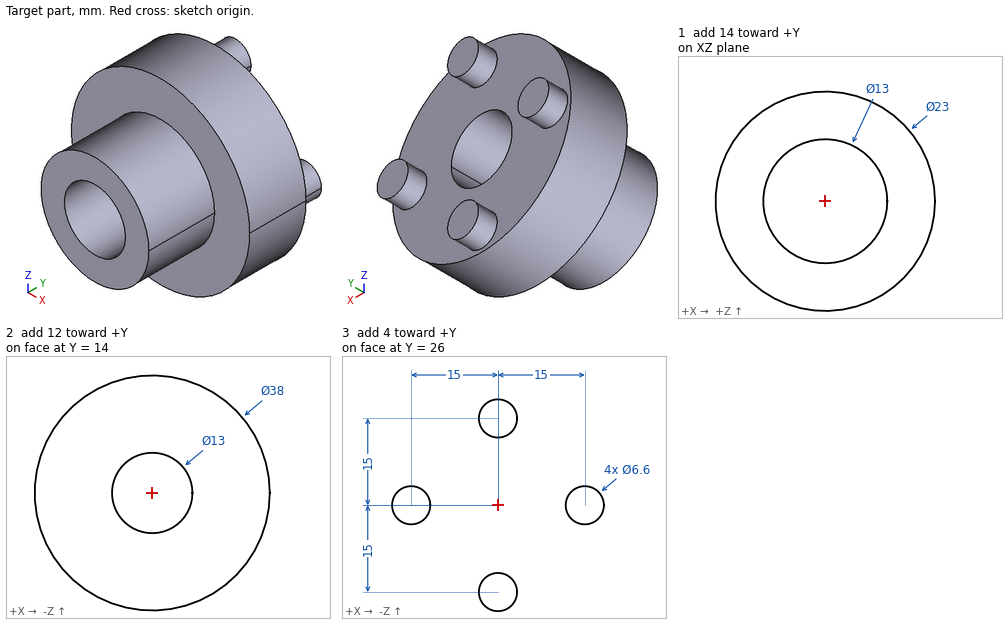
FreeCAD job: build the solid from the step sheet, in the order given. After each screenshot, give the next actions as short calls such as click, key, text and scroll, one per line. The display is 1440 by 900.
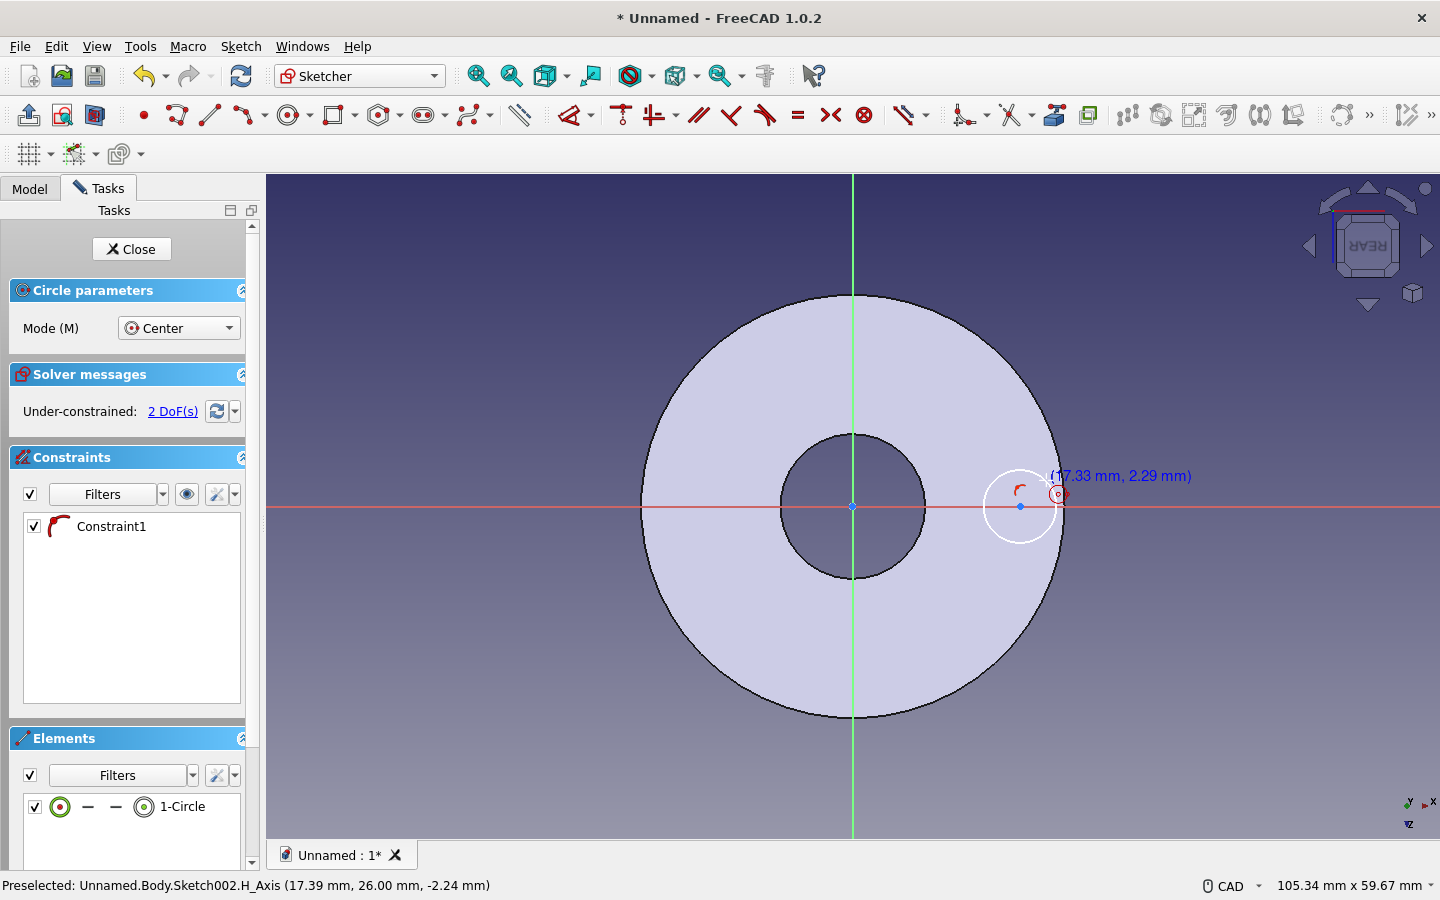
click(853, 339)
click(879, 313)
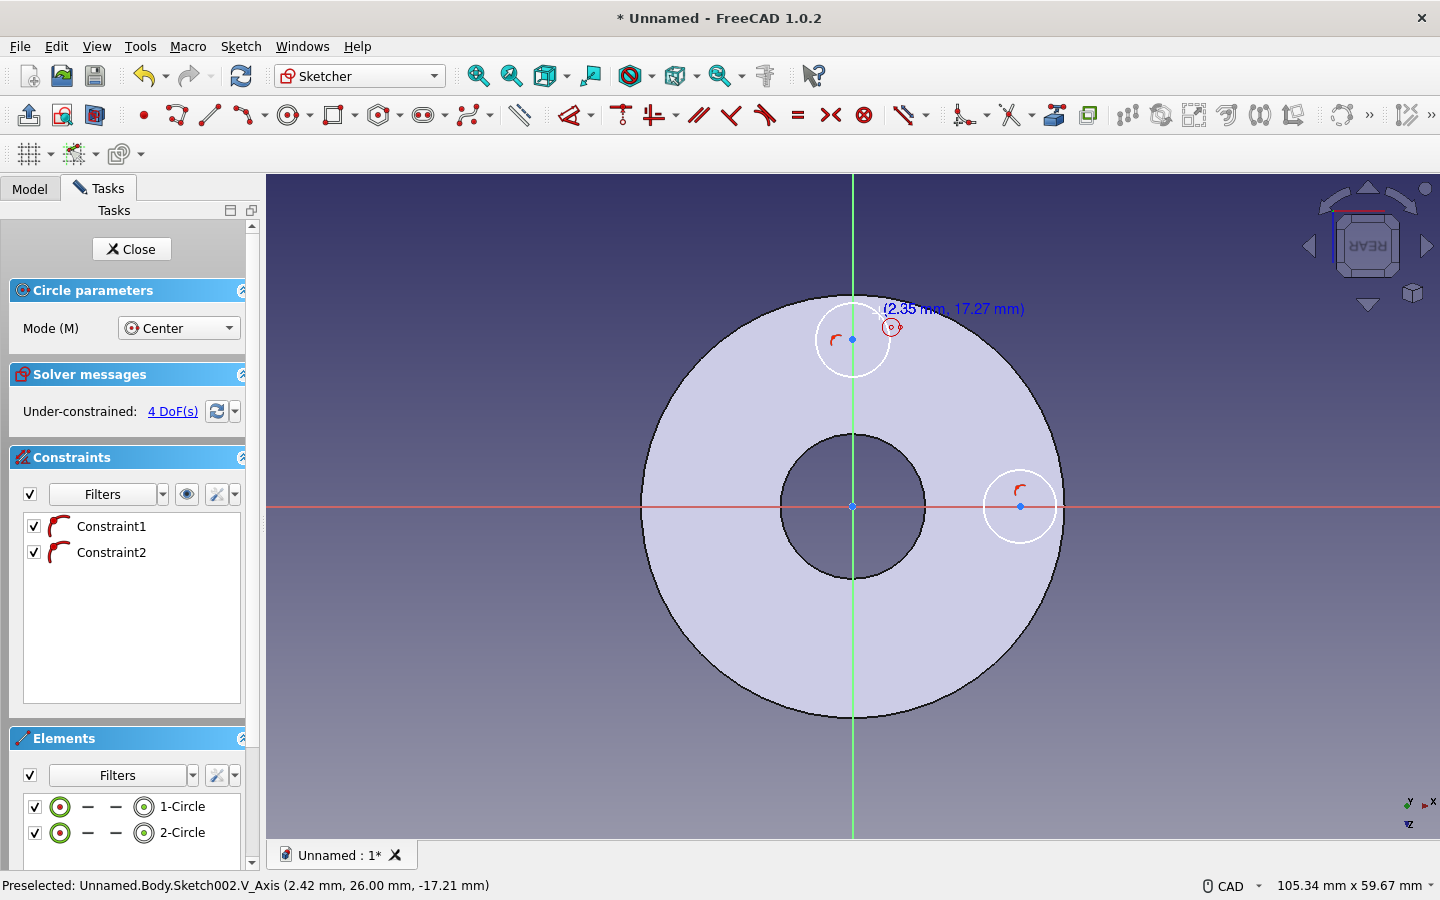
click(853, 674)
click(879, 648)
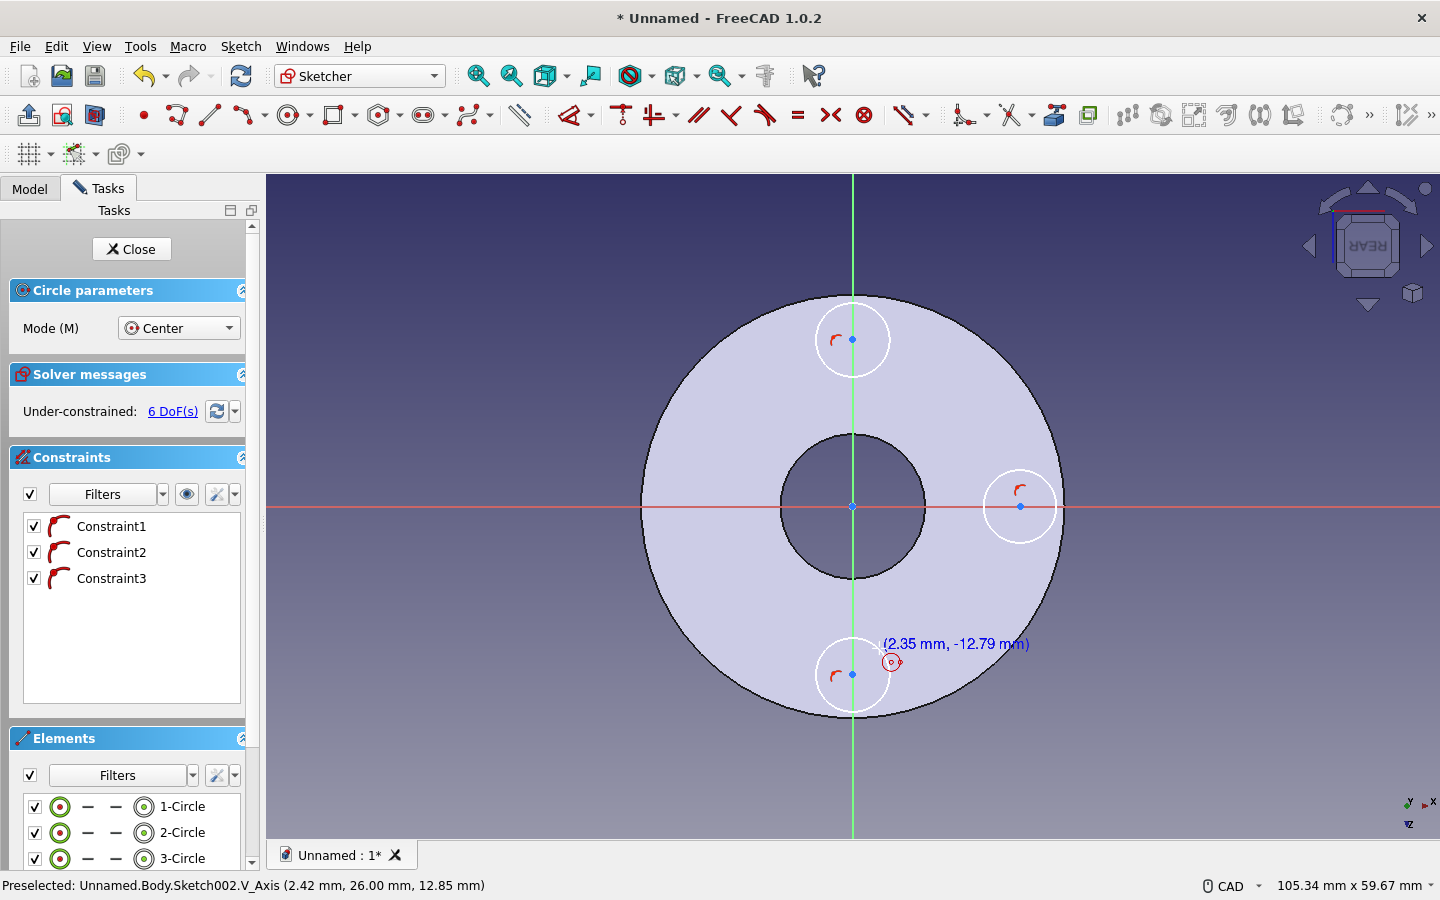
click(686, 506)
click(712, 480)
key(Escape)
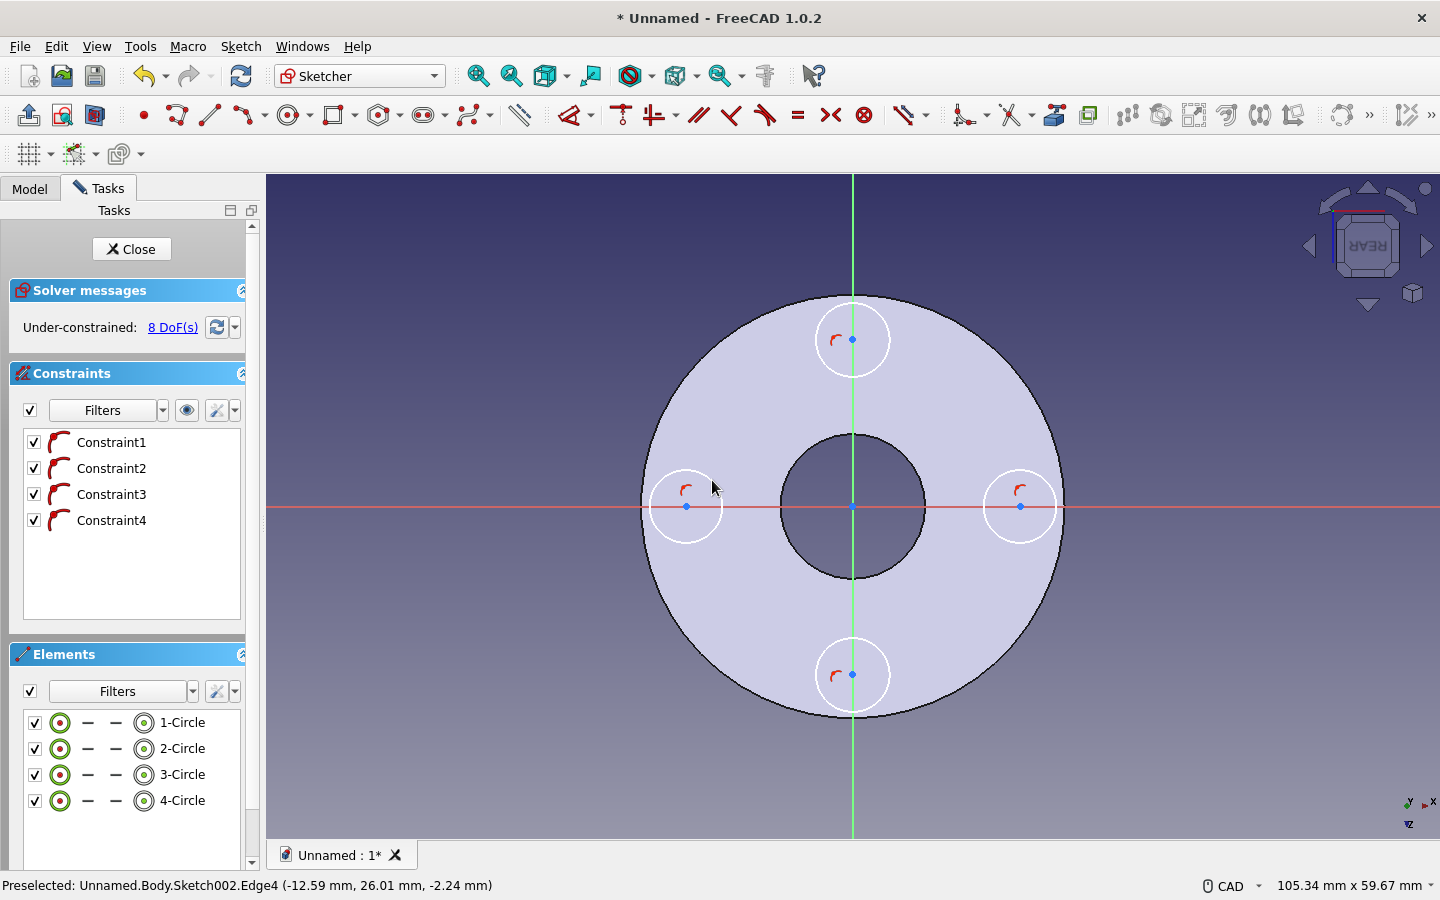
click(1046, 481)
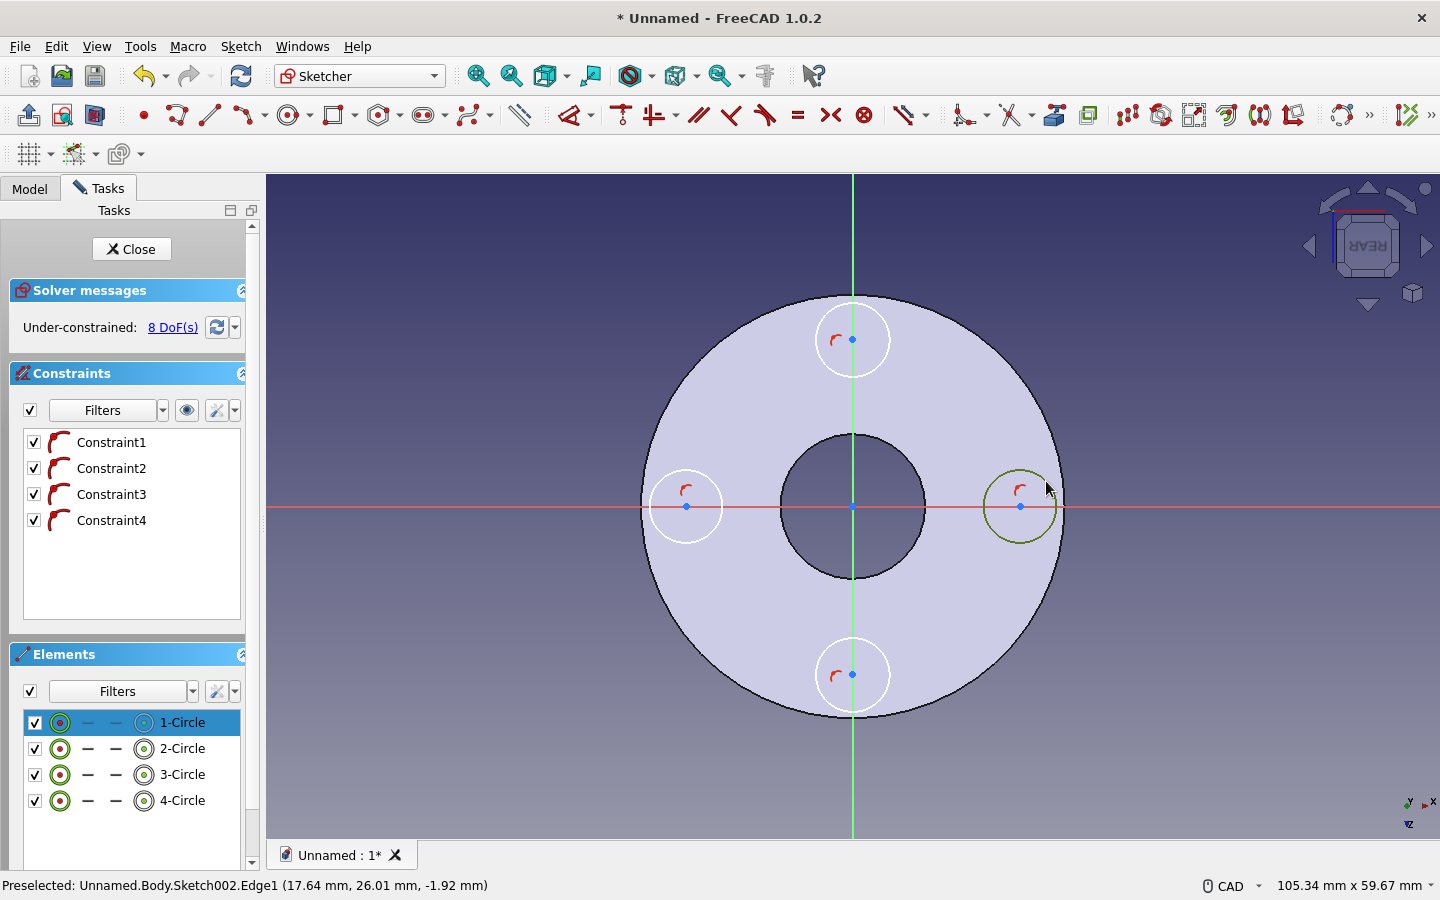
click(879, 314)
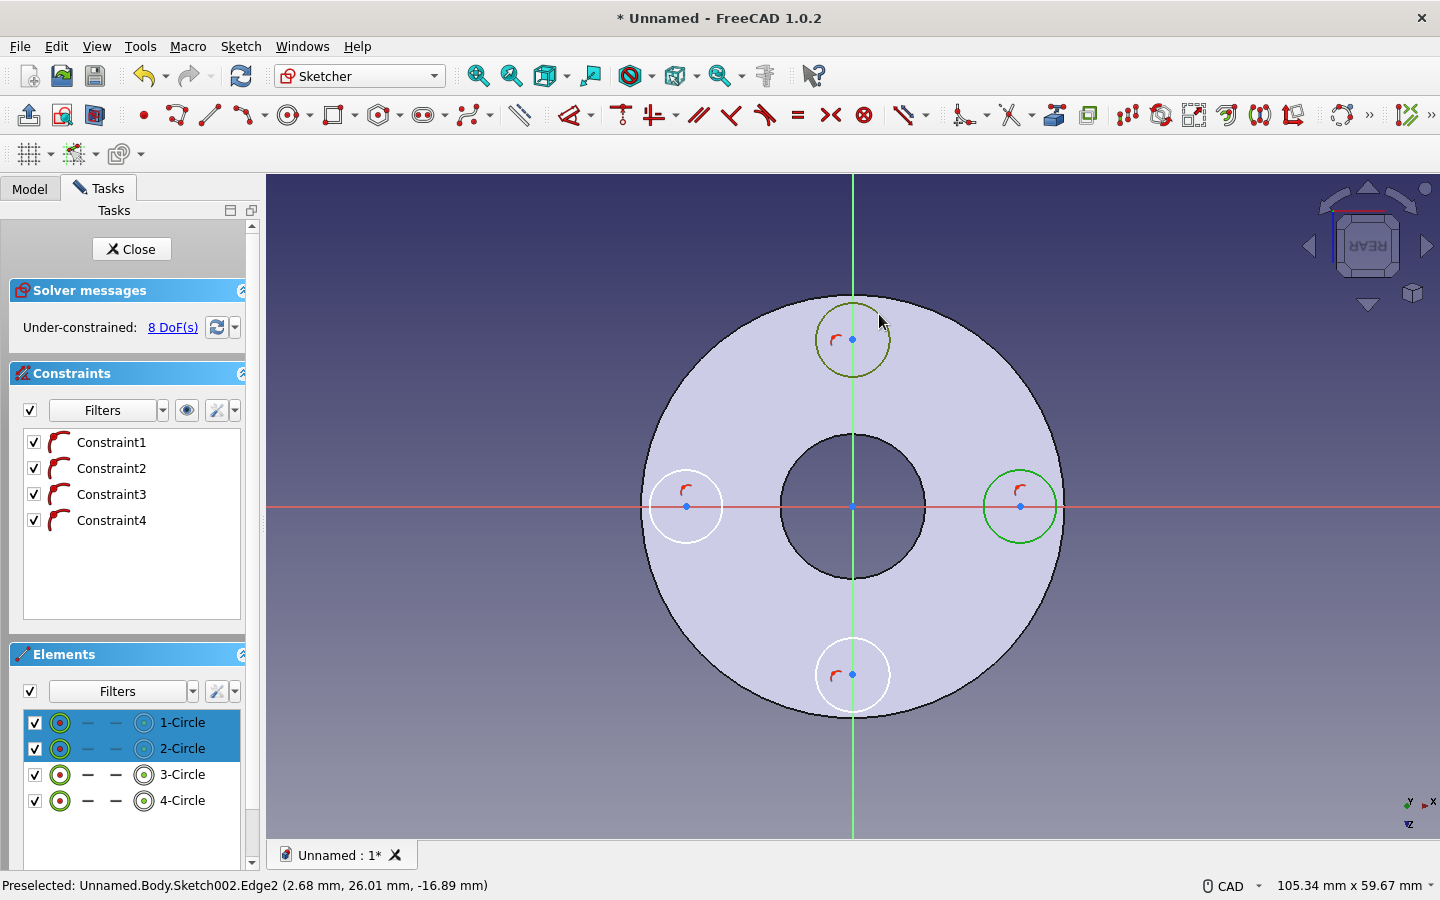
click(879, 649)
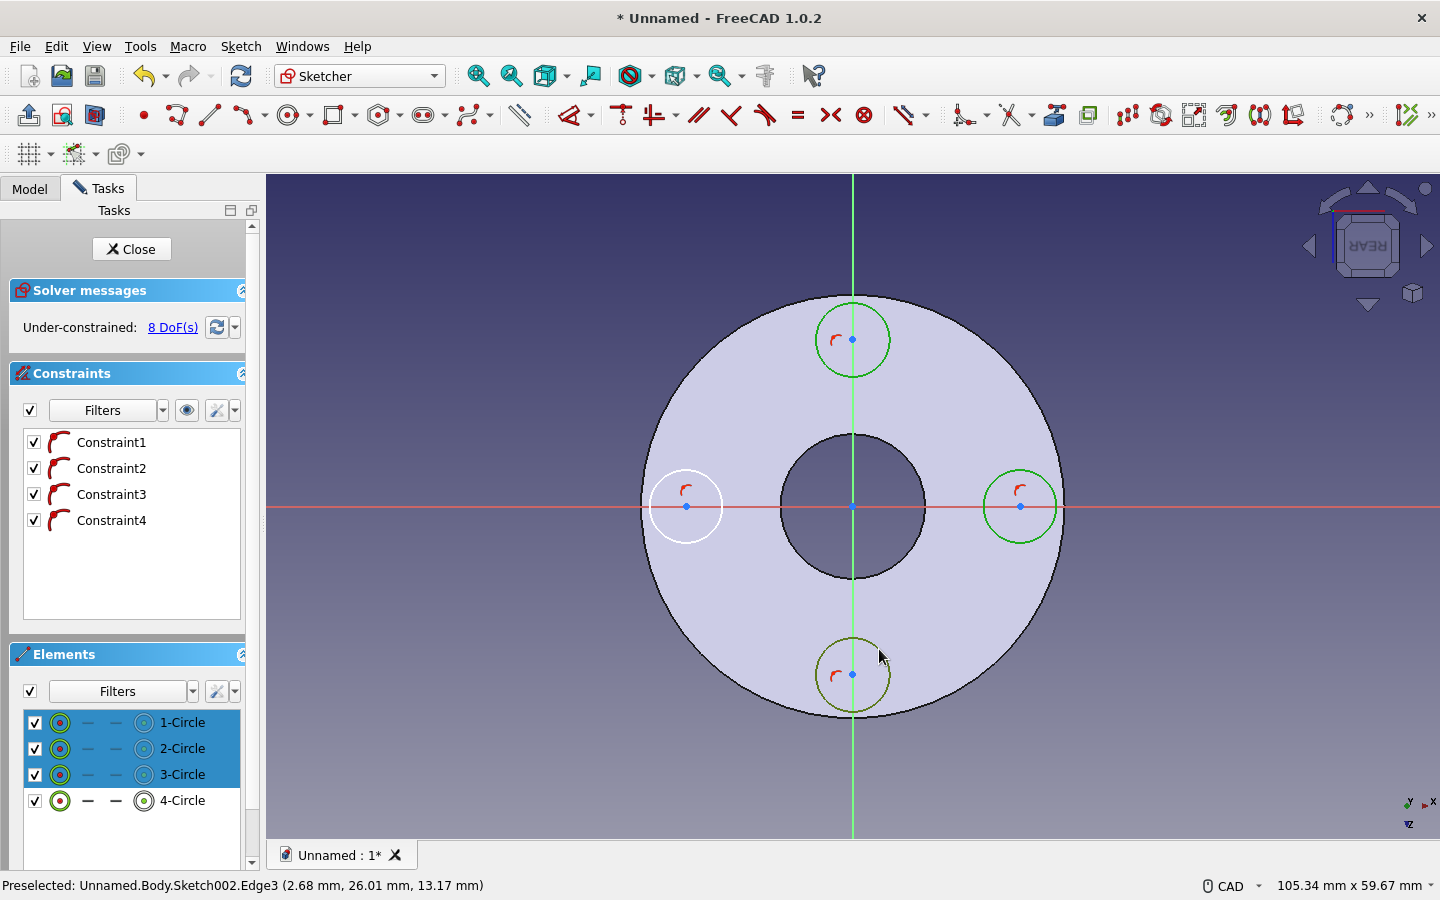
click(712, 481)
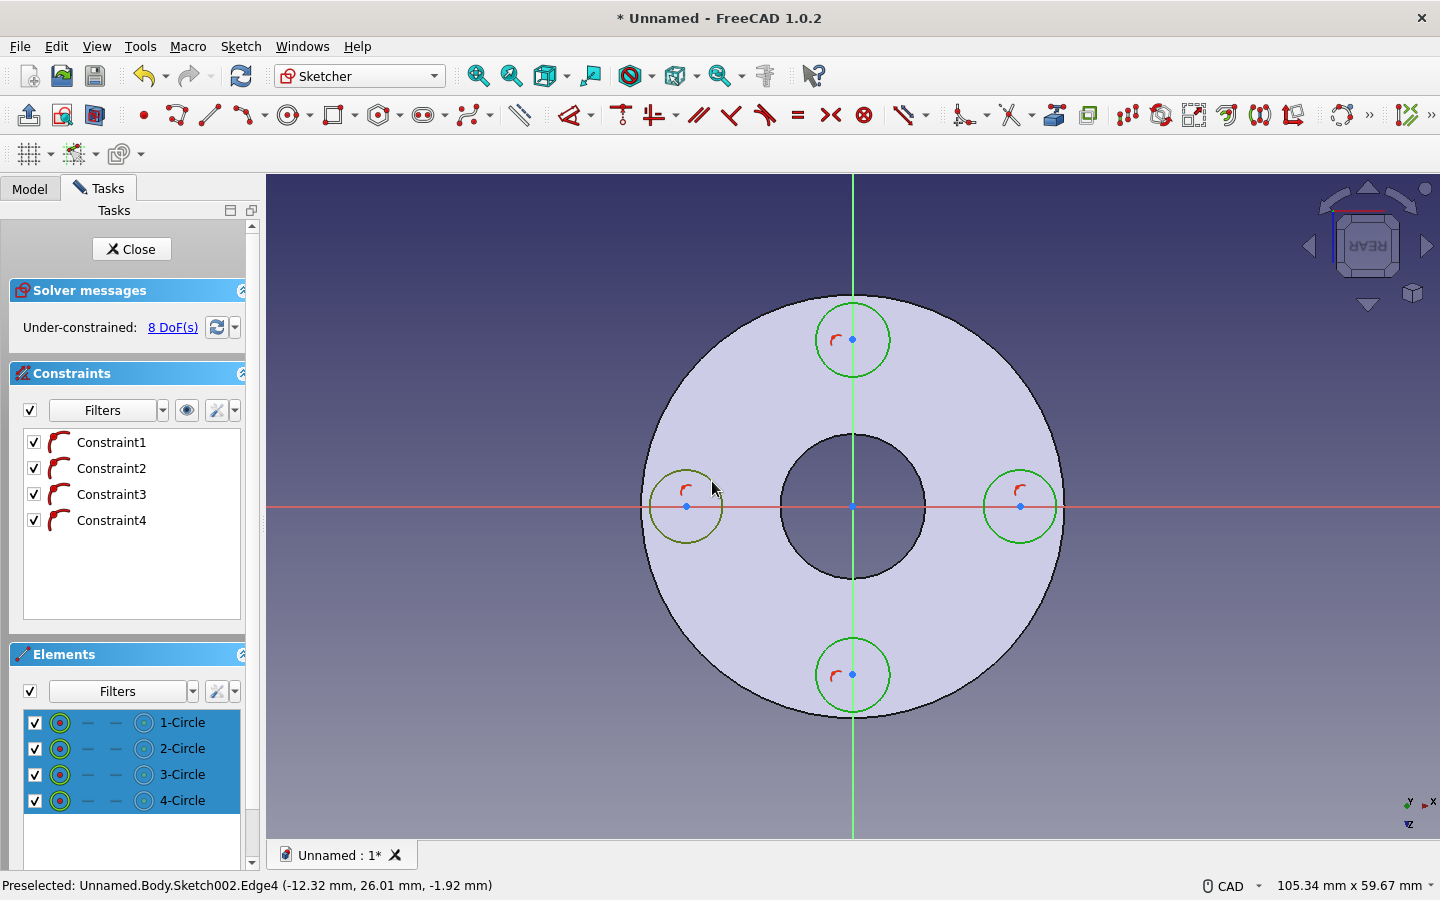
click(798, 116)